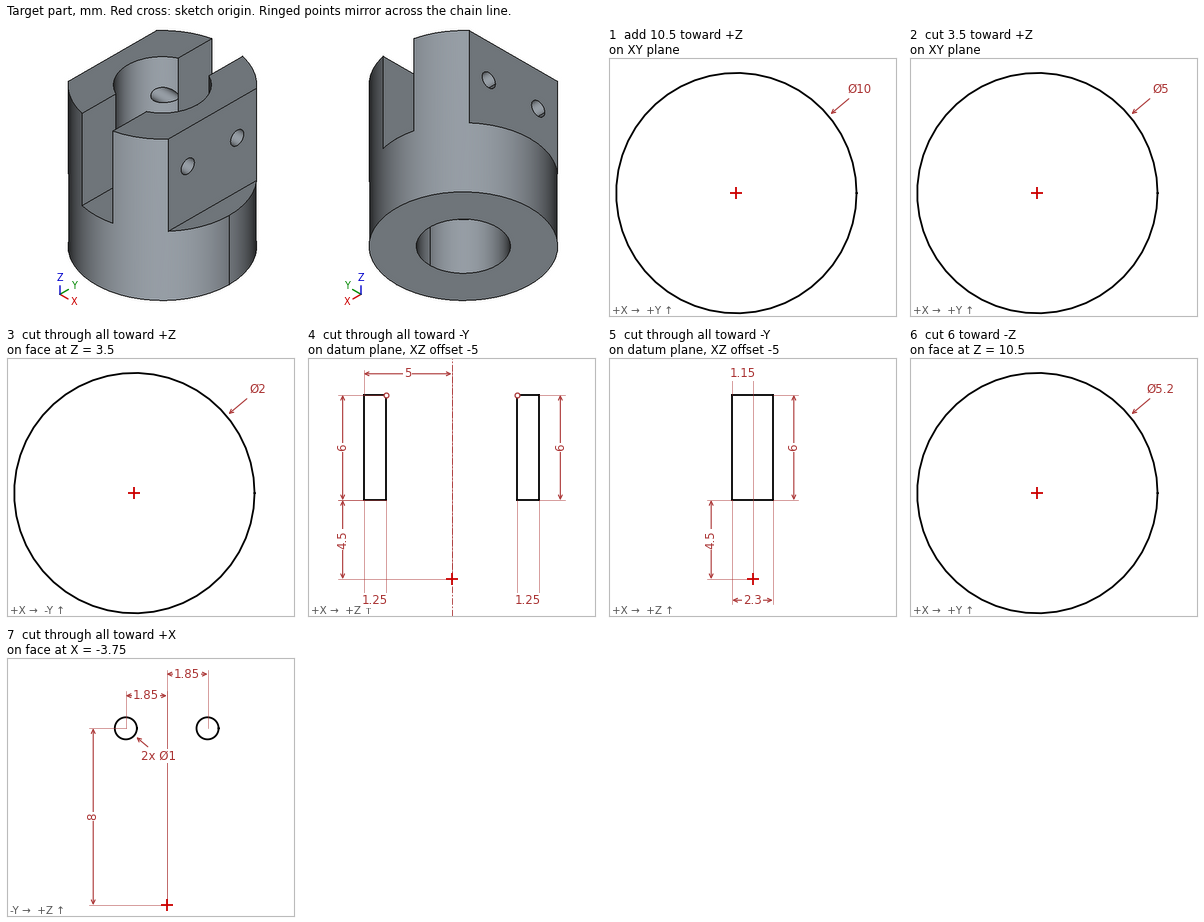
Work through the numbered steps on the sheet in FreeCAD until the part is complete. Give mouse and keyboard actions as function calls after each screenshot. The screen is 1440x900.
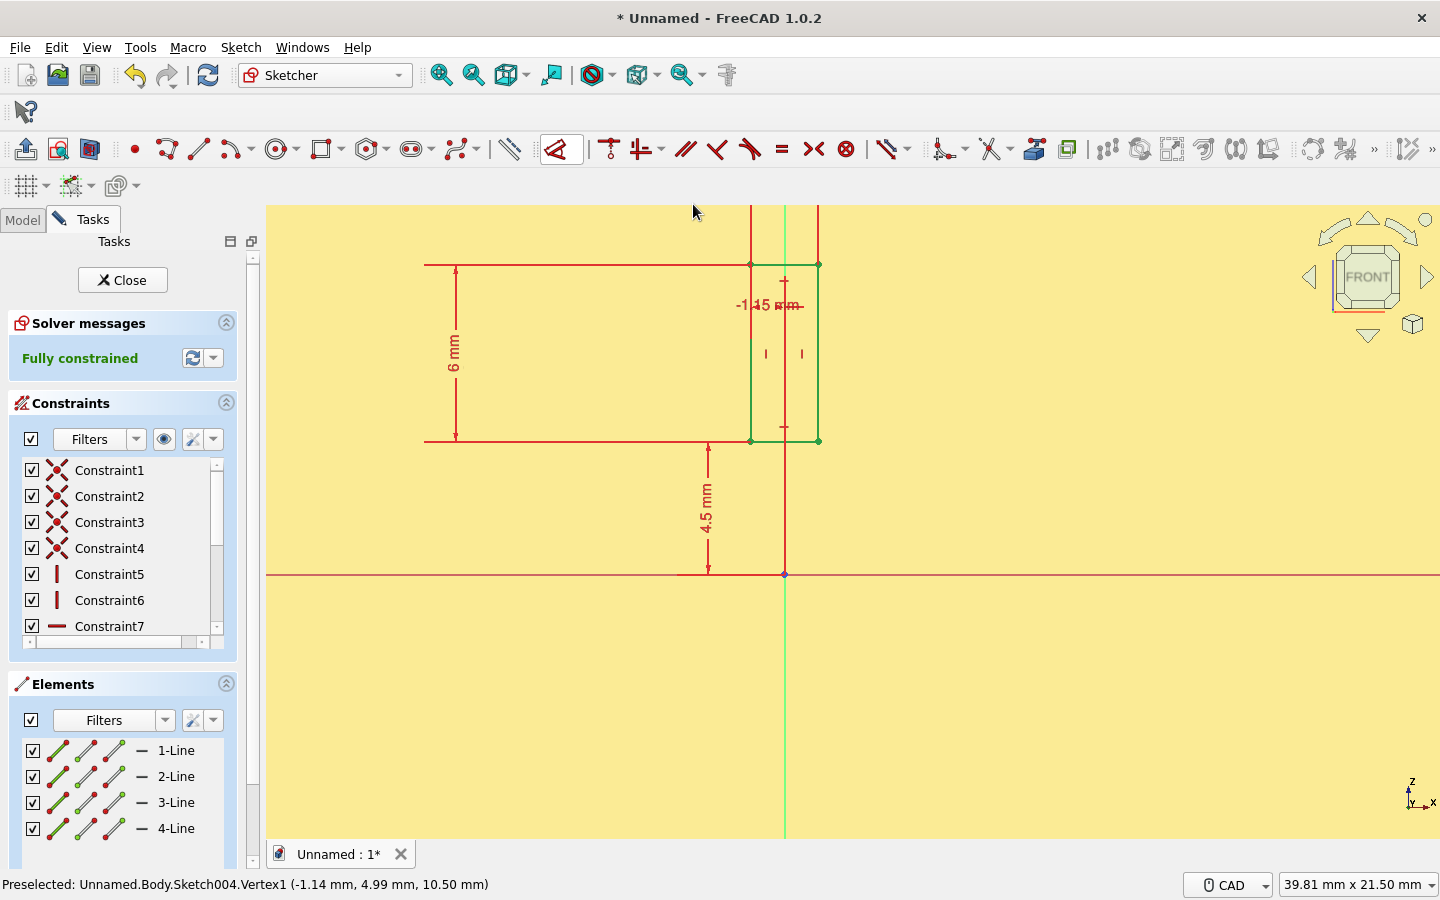
click(123, 280)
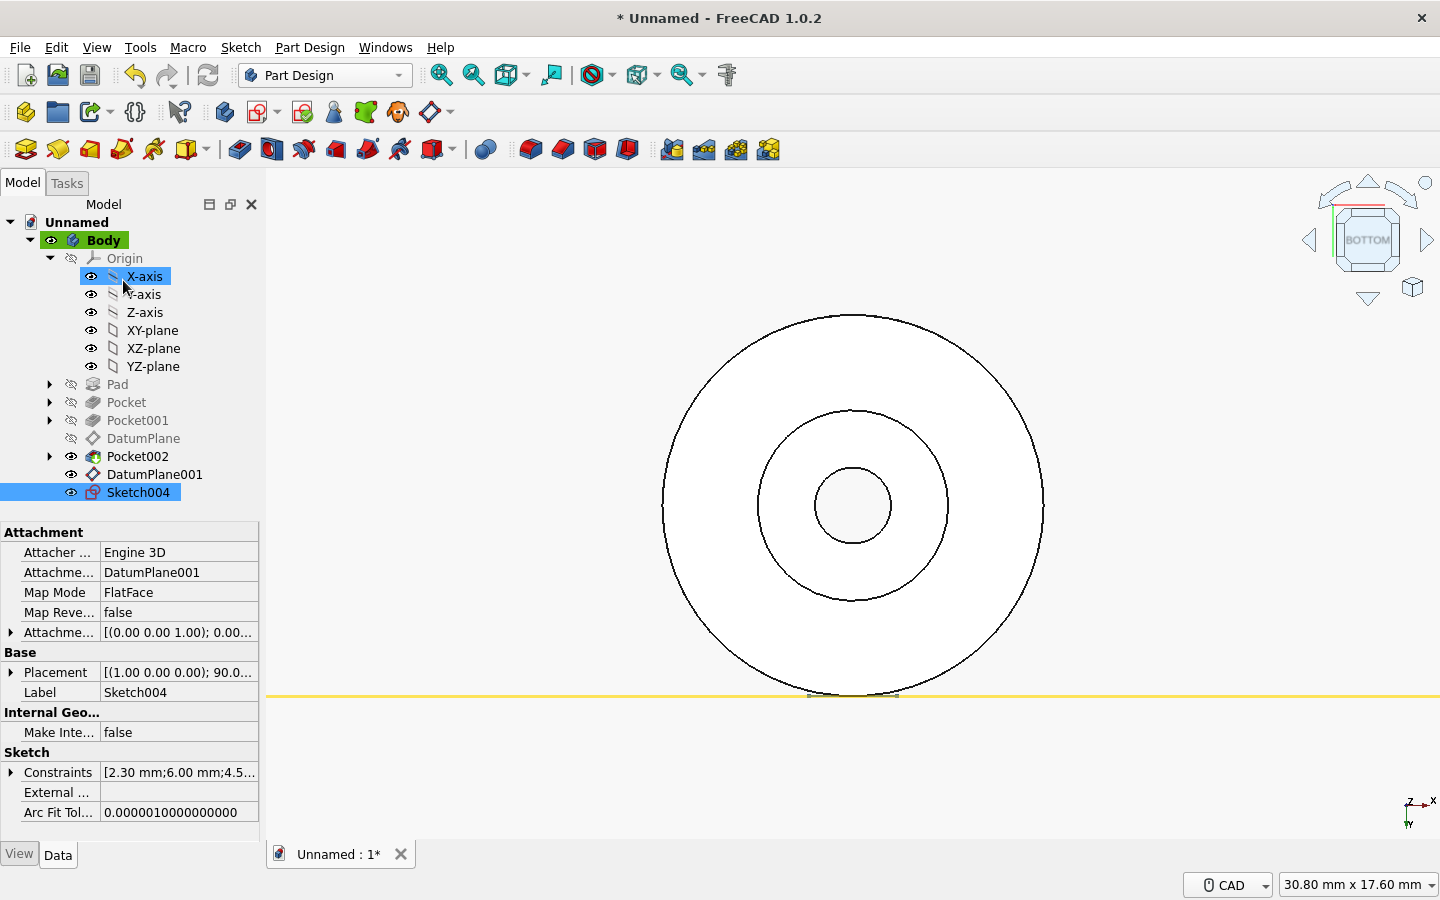
click(240, 150)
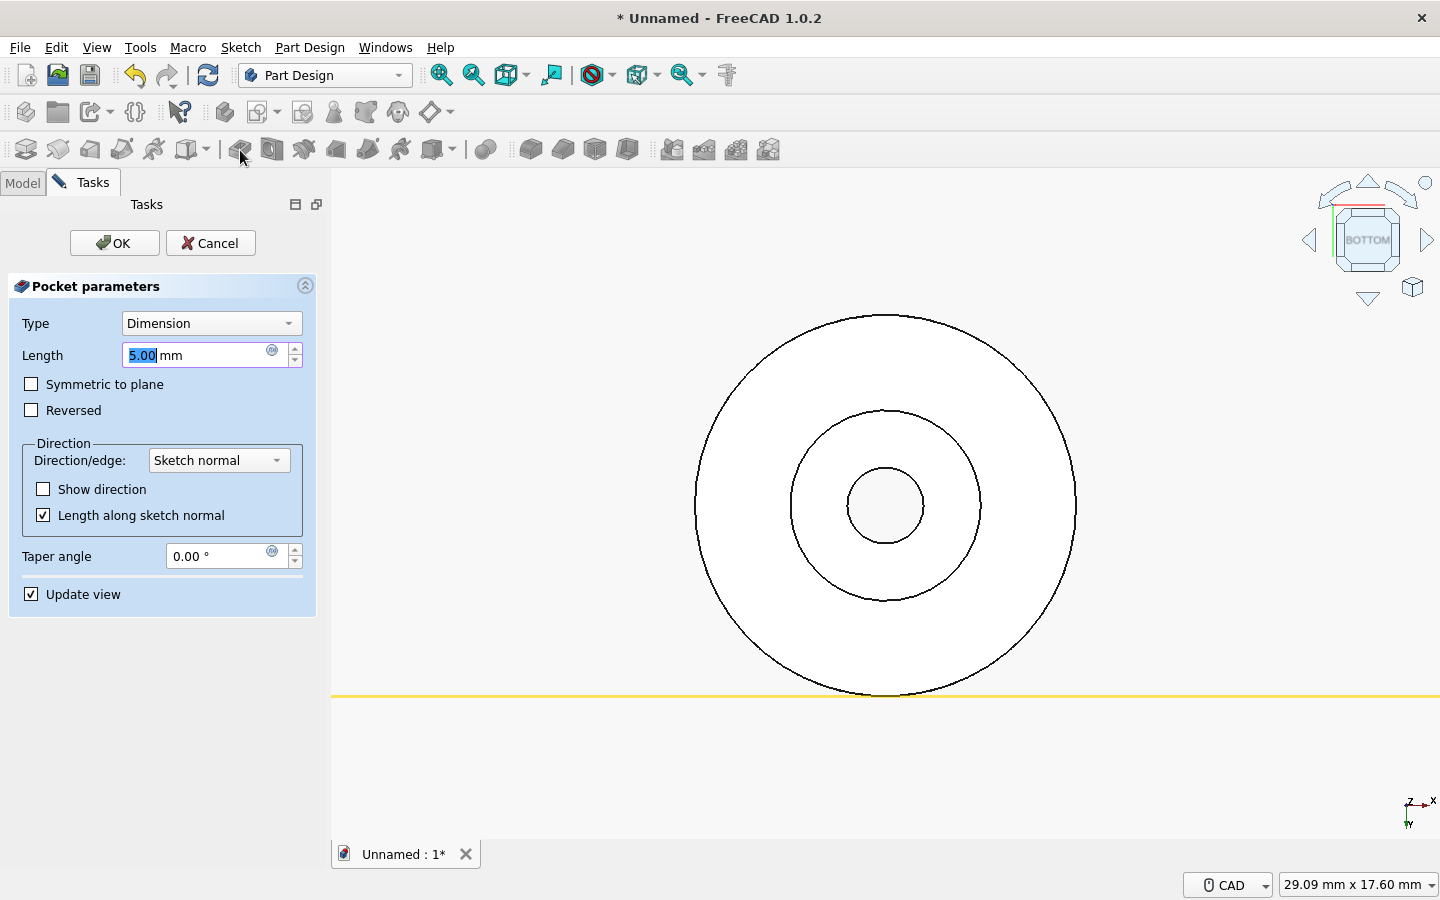
click(212, 324)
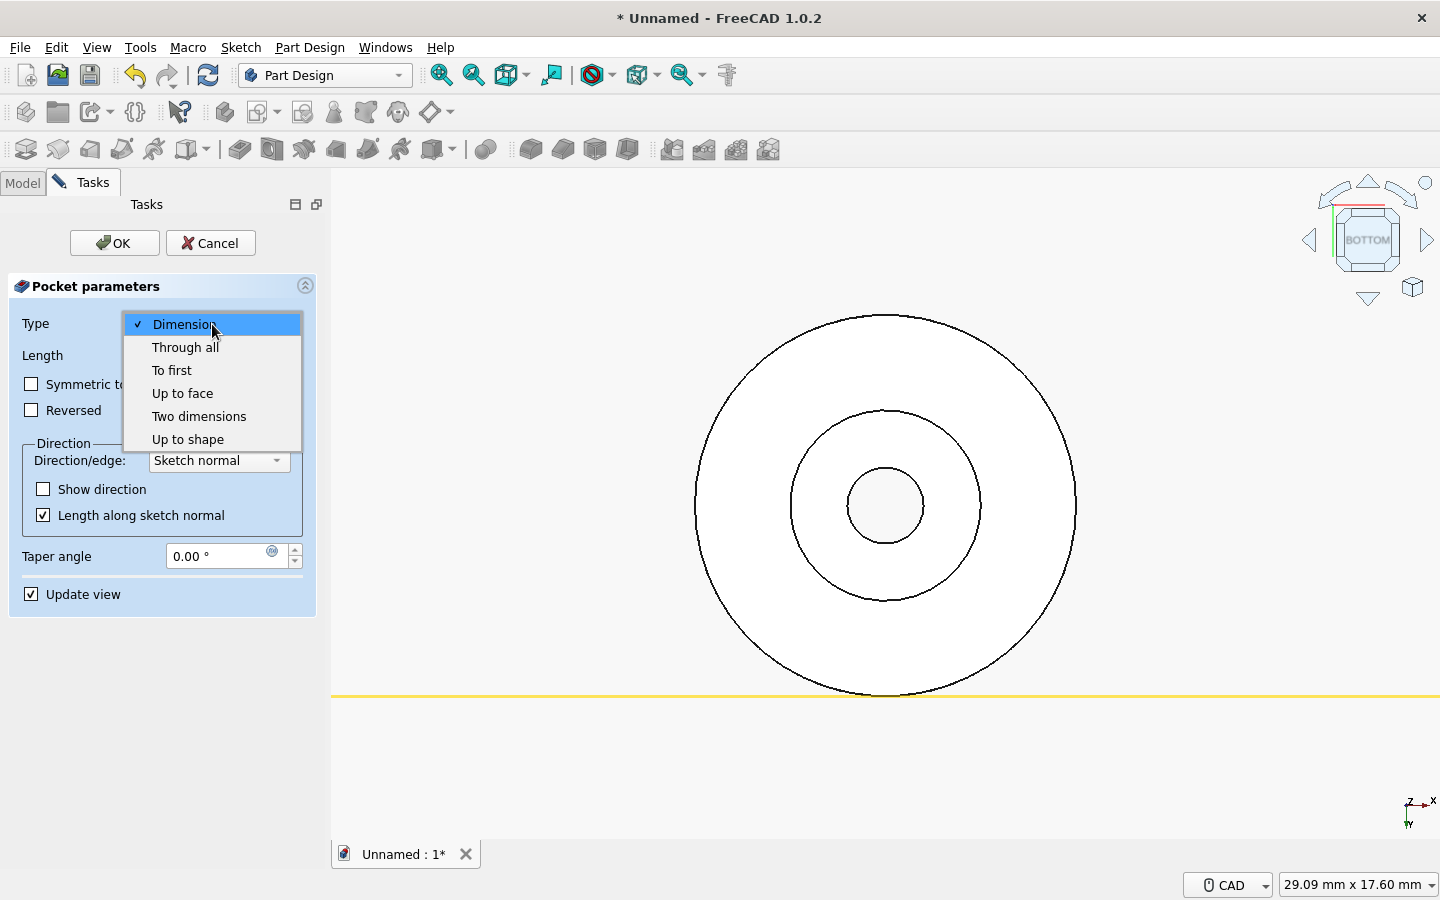
click(212, 348)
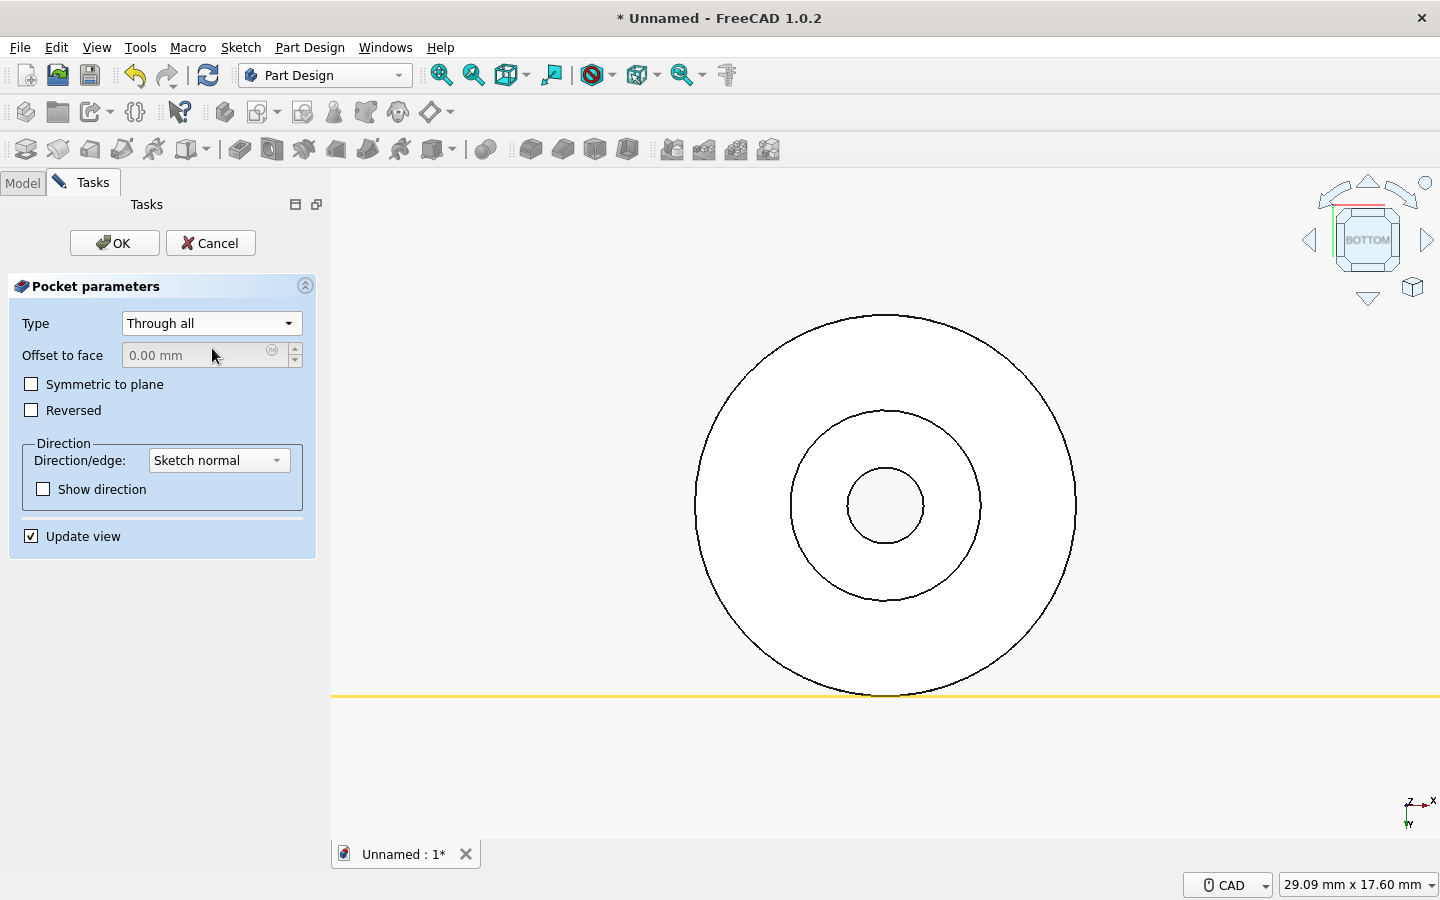
click(30, 410)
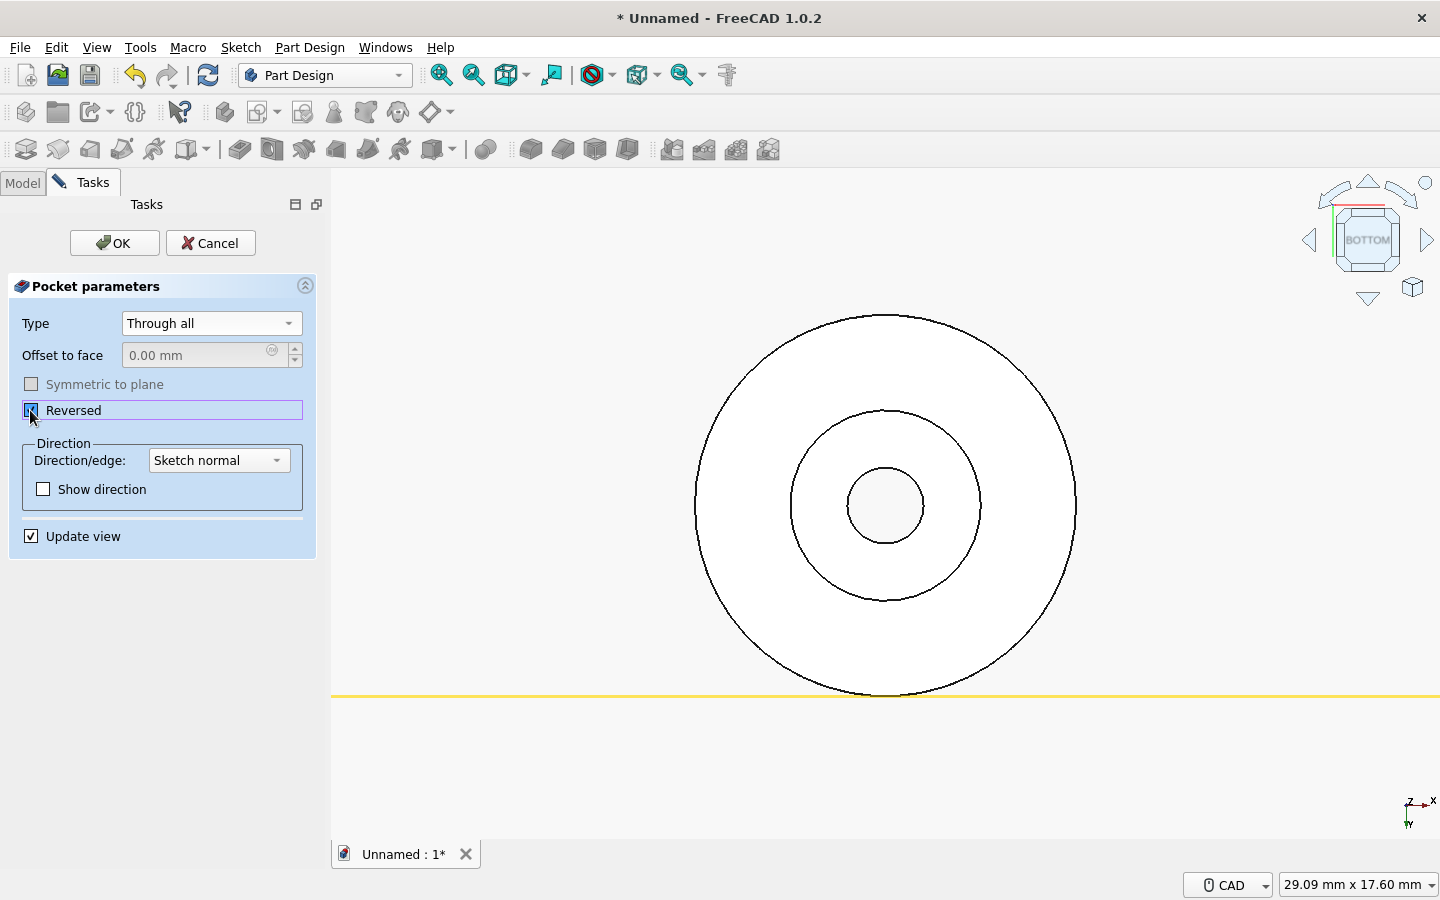
click(115, 243)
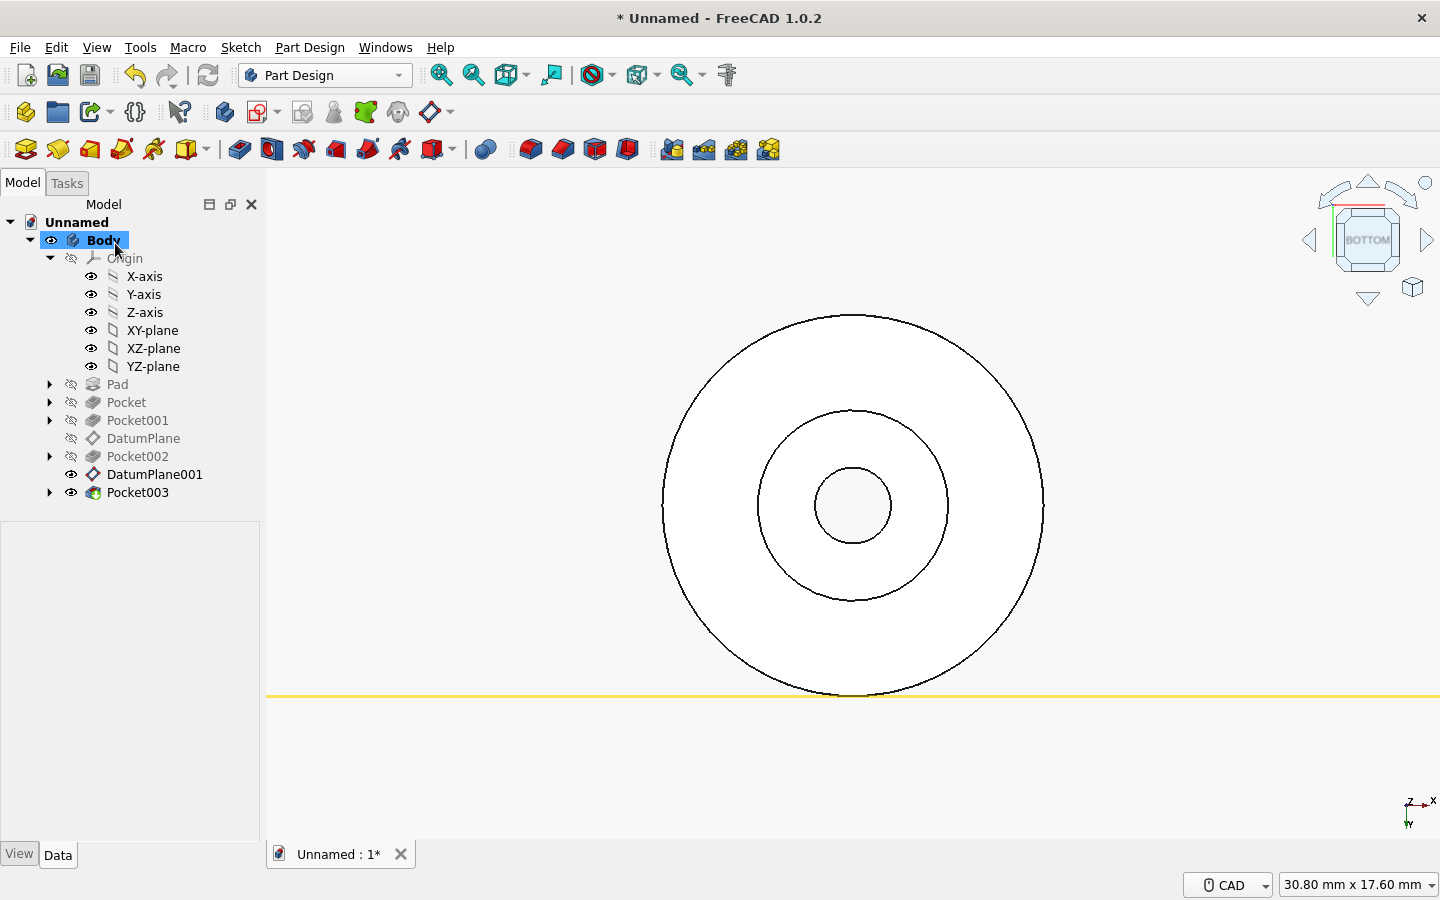
click(116, 474)
key(space)